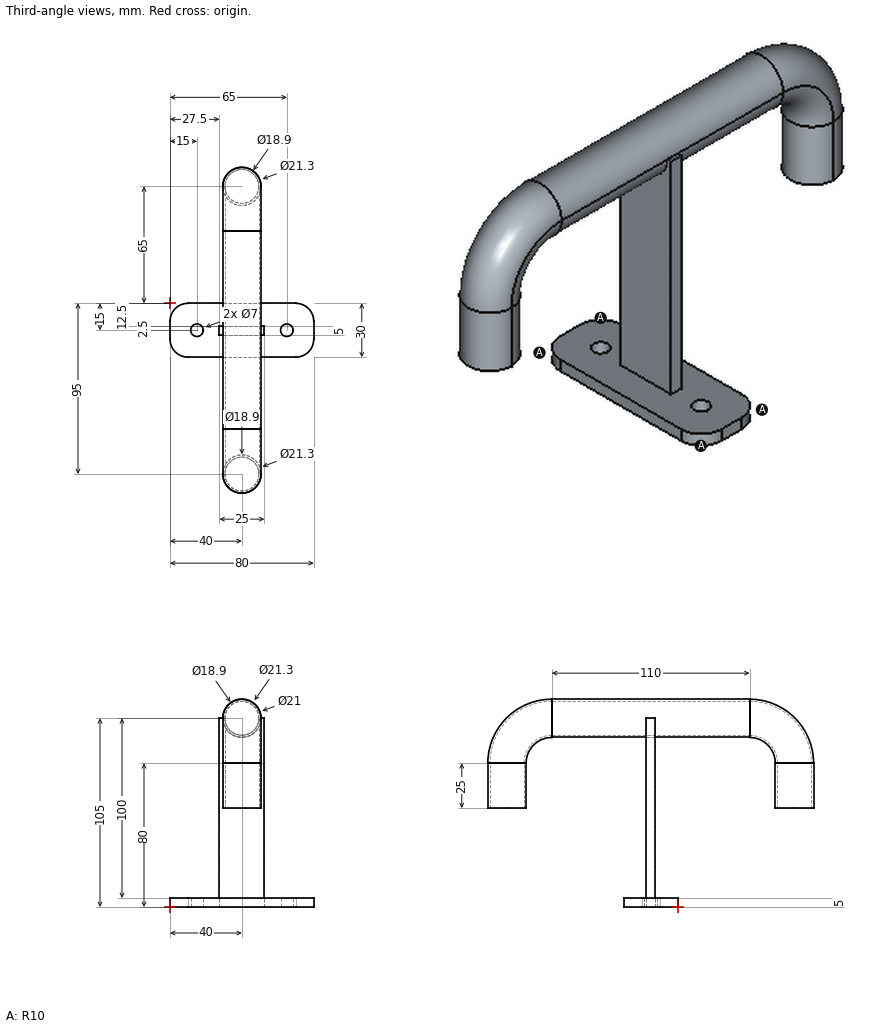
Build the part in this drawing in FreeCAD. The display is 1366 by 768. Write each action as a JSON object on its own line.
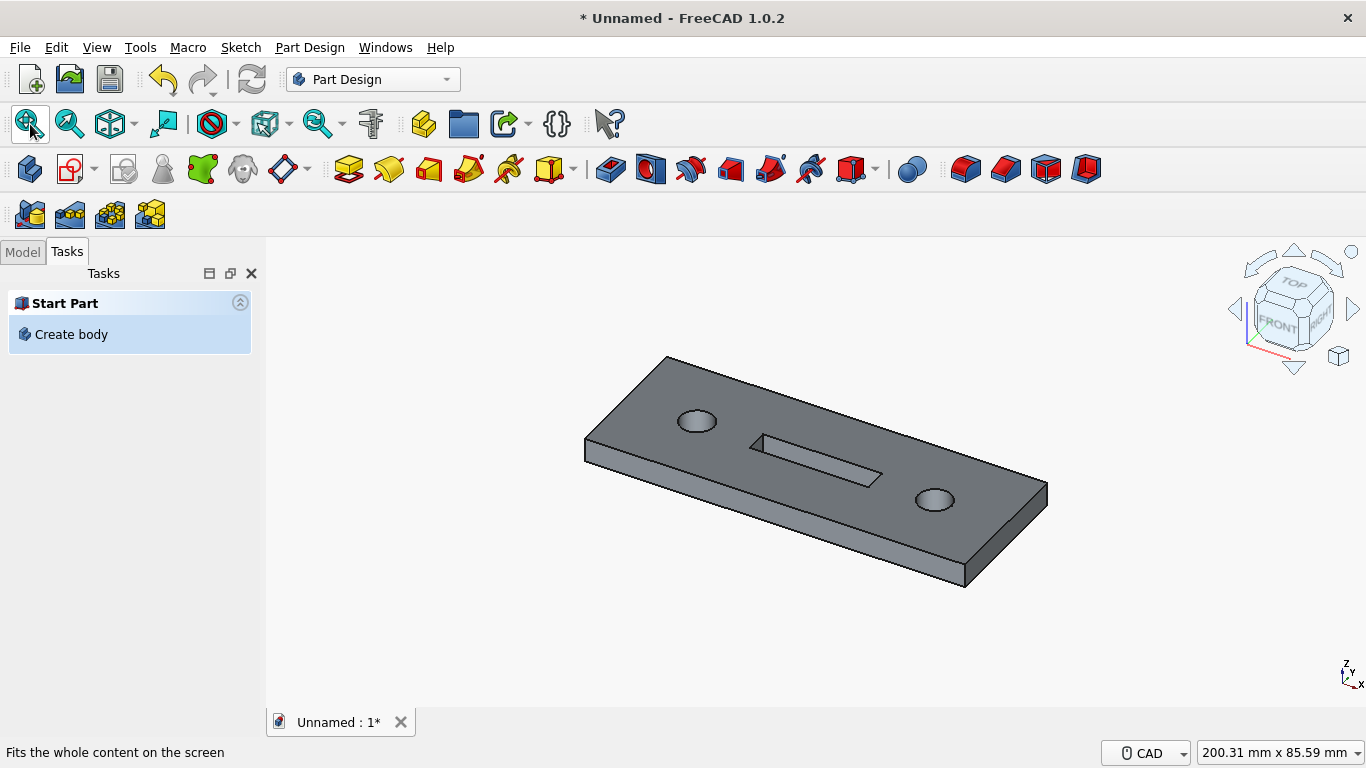
{"action": "left_click", "coordinate": [965, 575]}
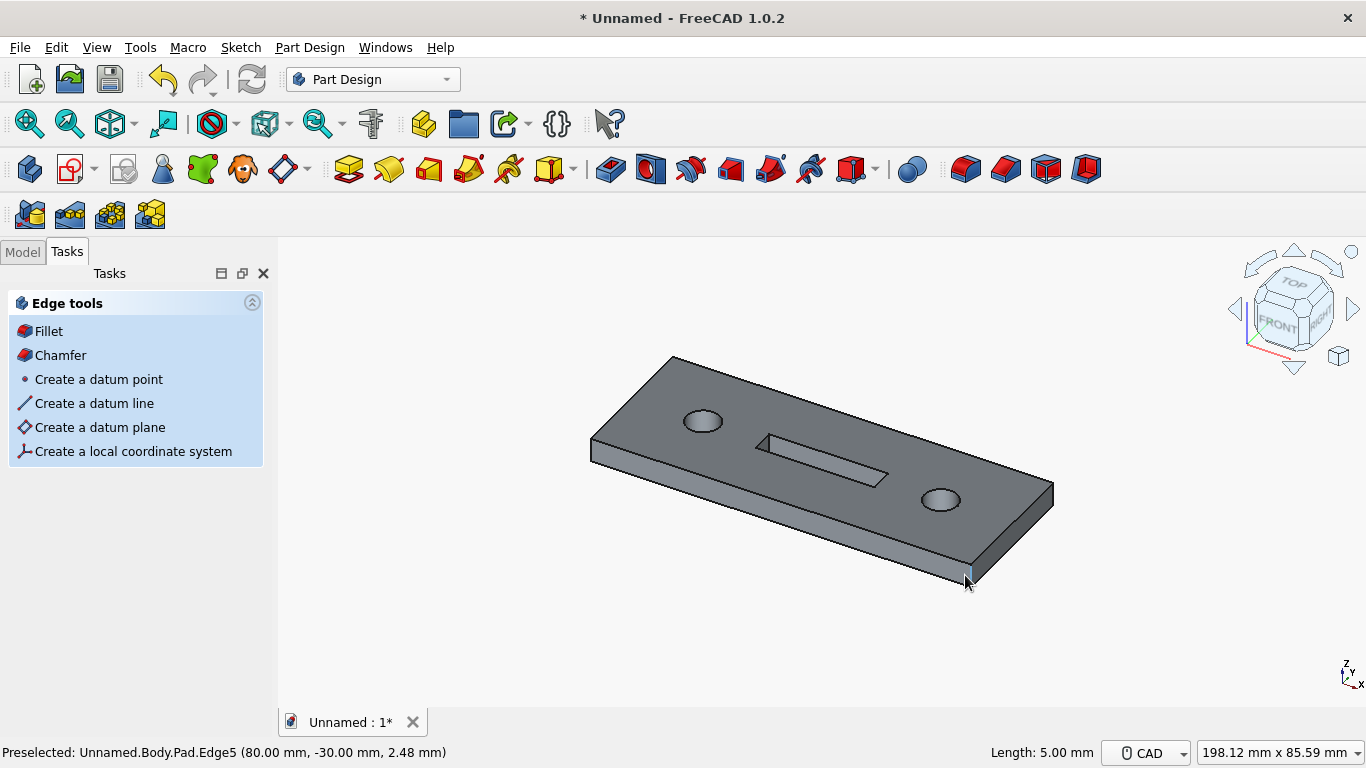
{"action": "key", "text": "0"}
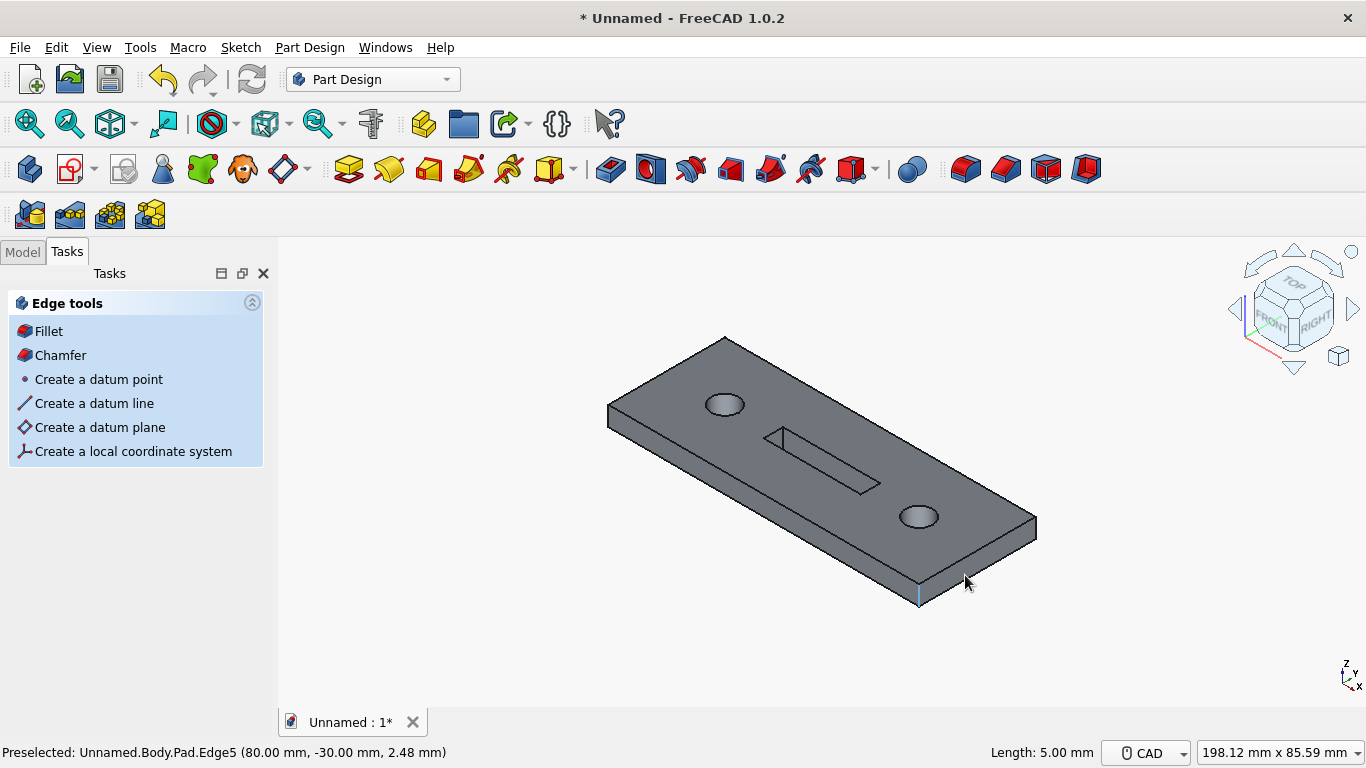
{"action": "key", "text": "2"}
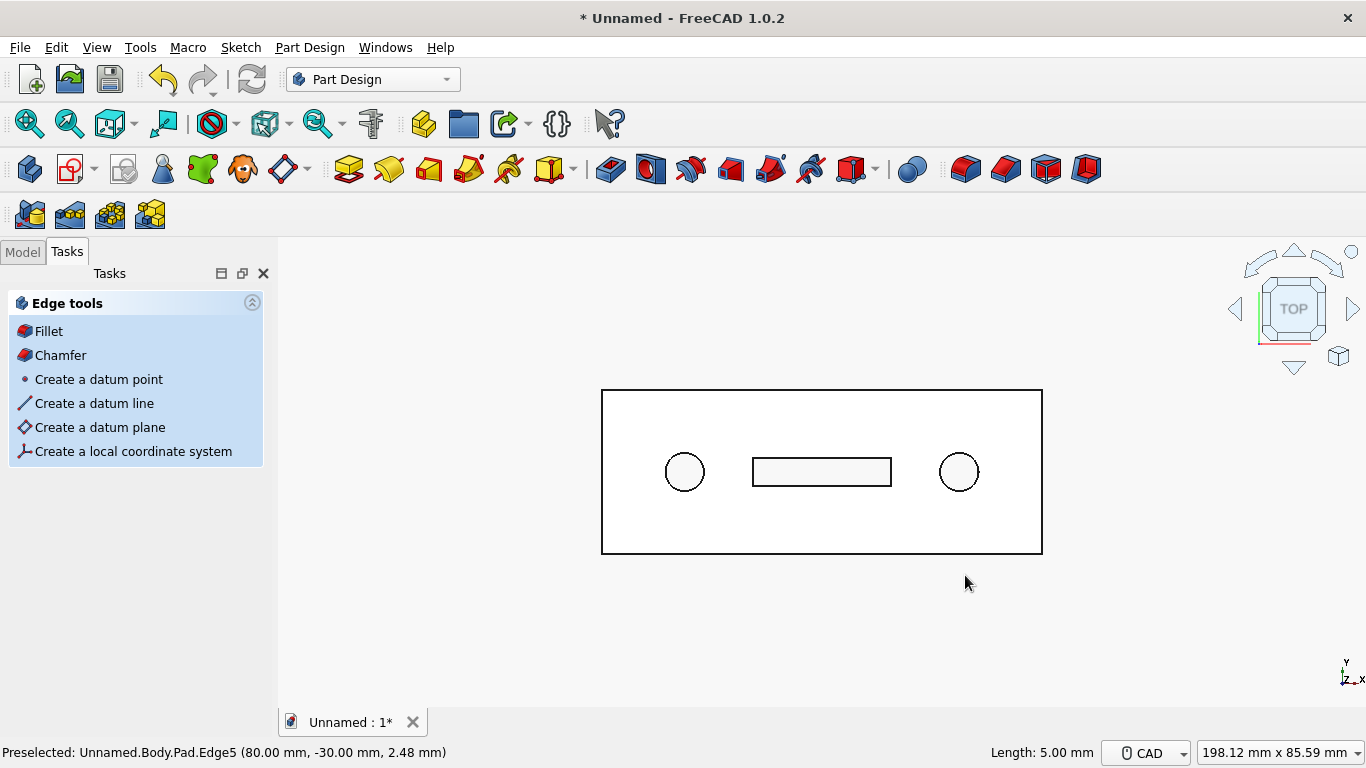
{"action": "left_click", "coordinate": [30, 124]}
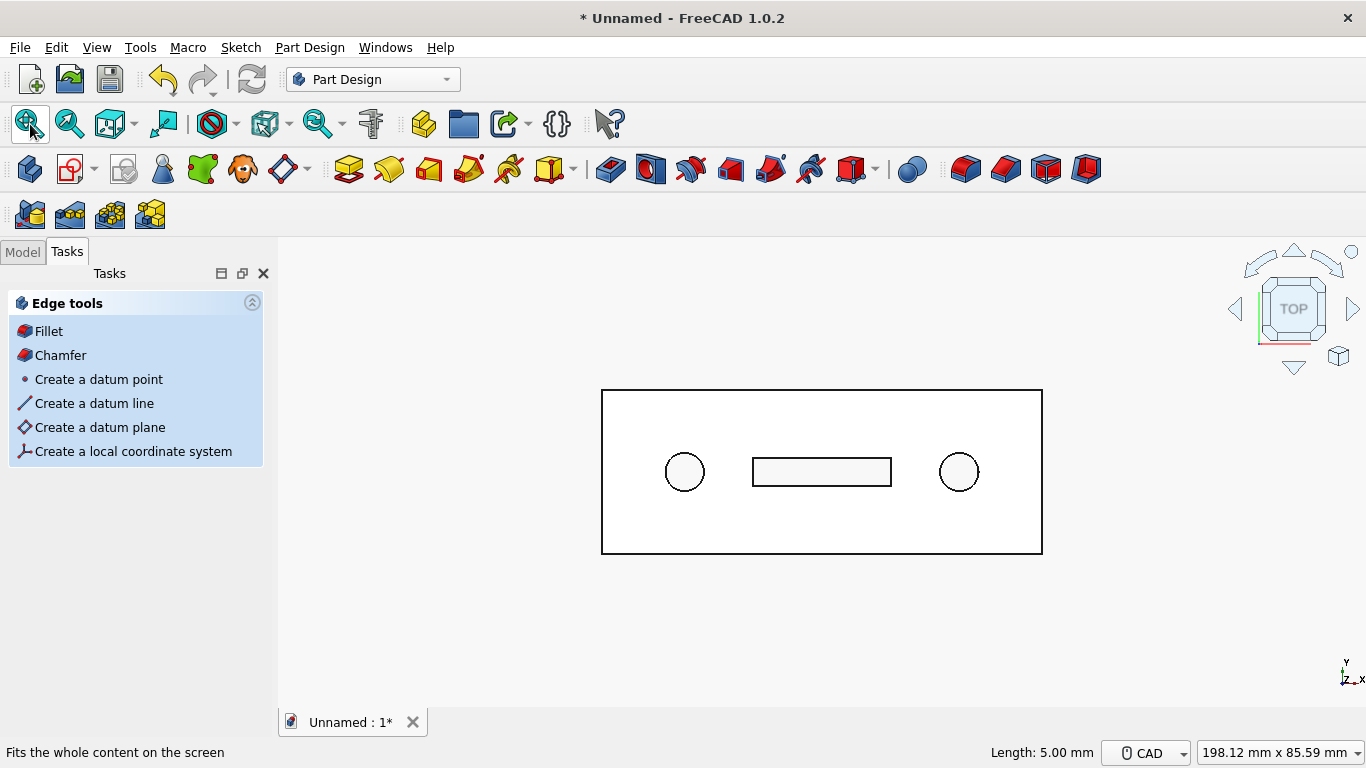
{"action": "key", "text": "1"}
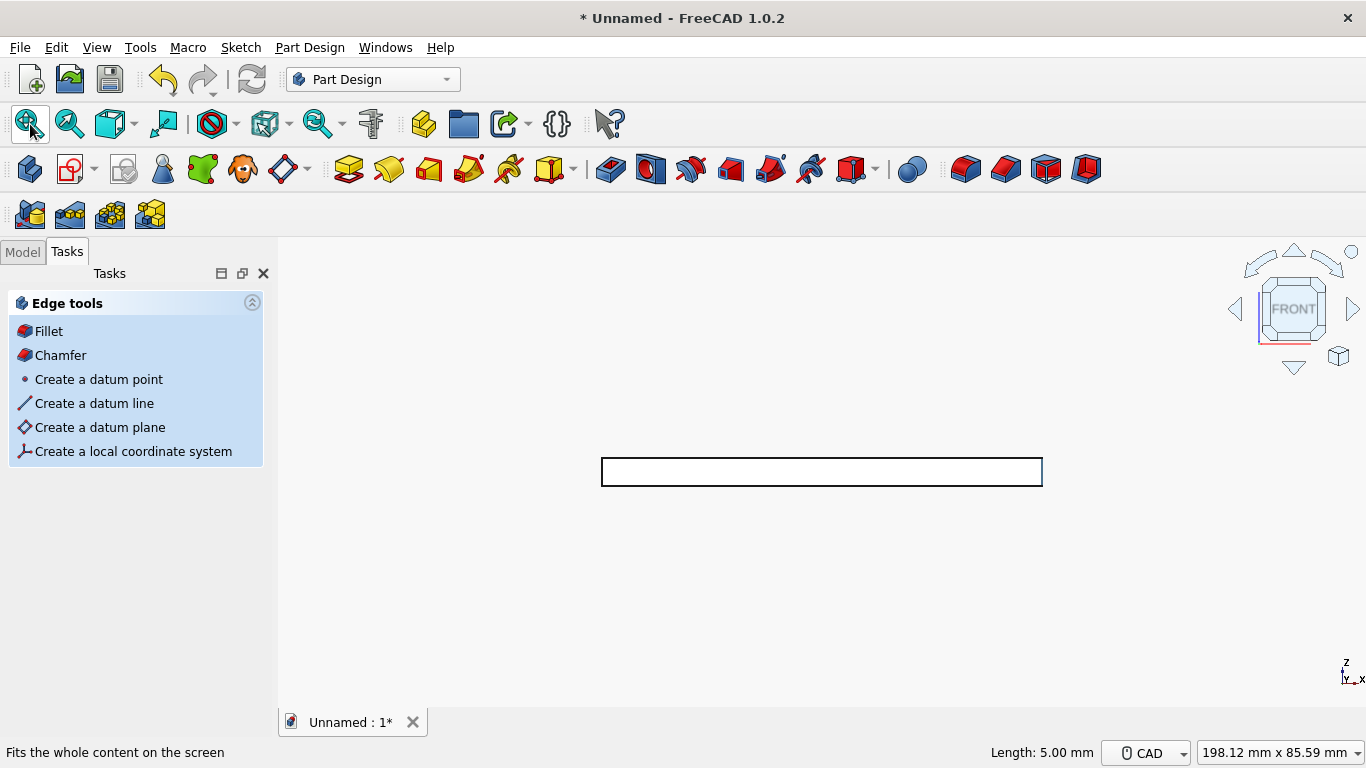
{"action": "left_click", "coordinate": [30, 124]}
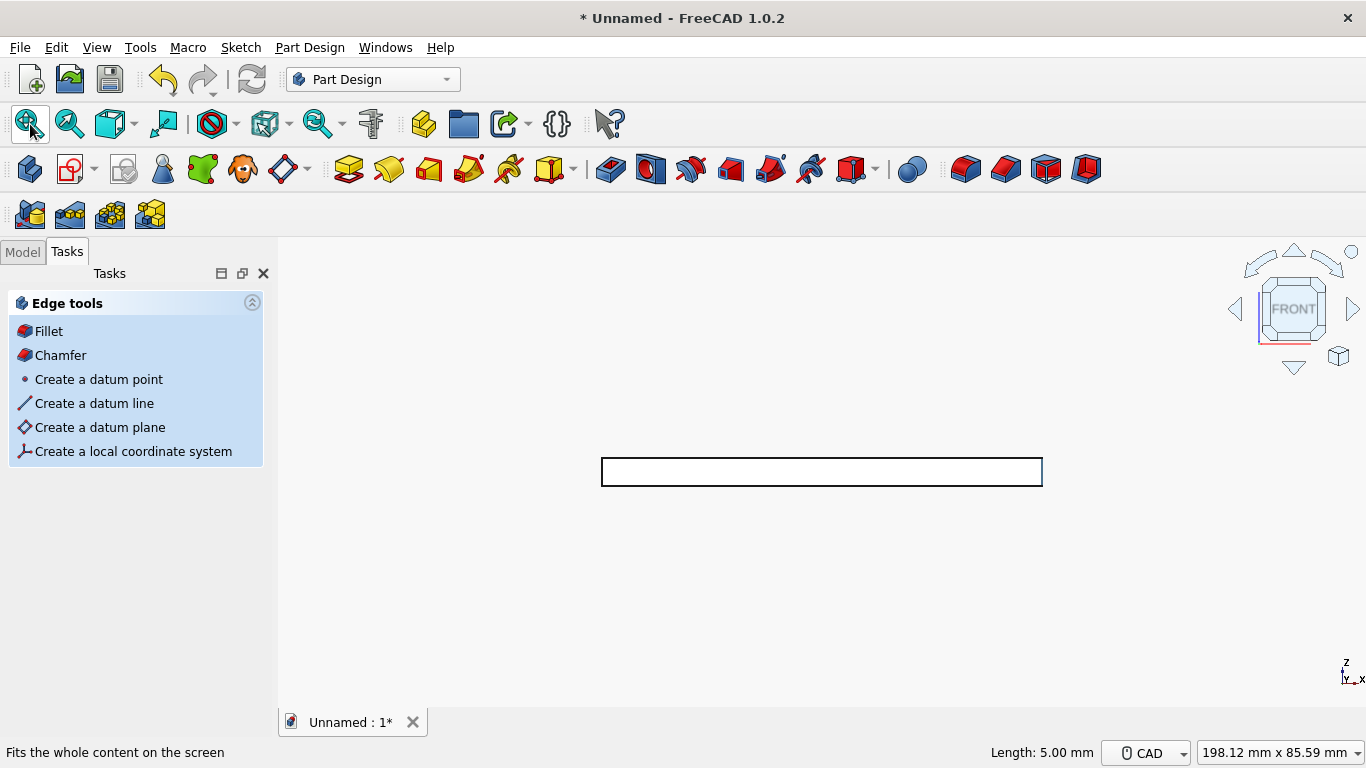
{"action": "left_click", "coordinate": [602, 471], "text": "ctrl"}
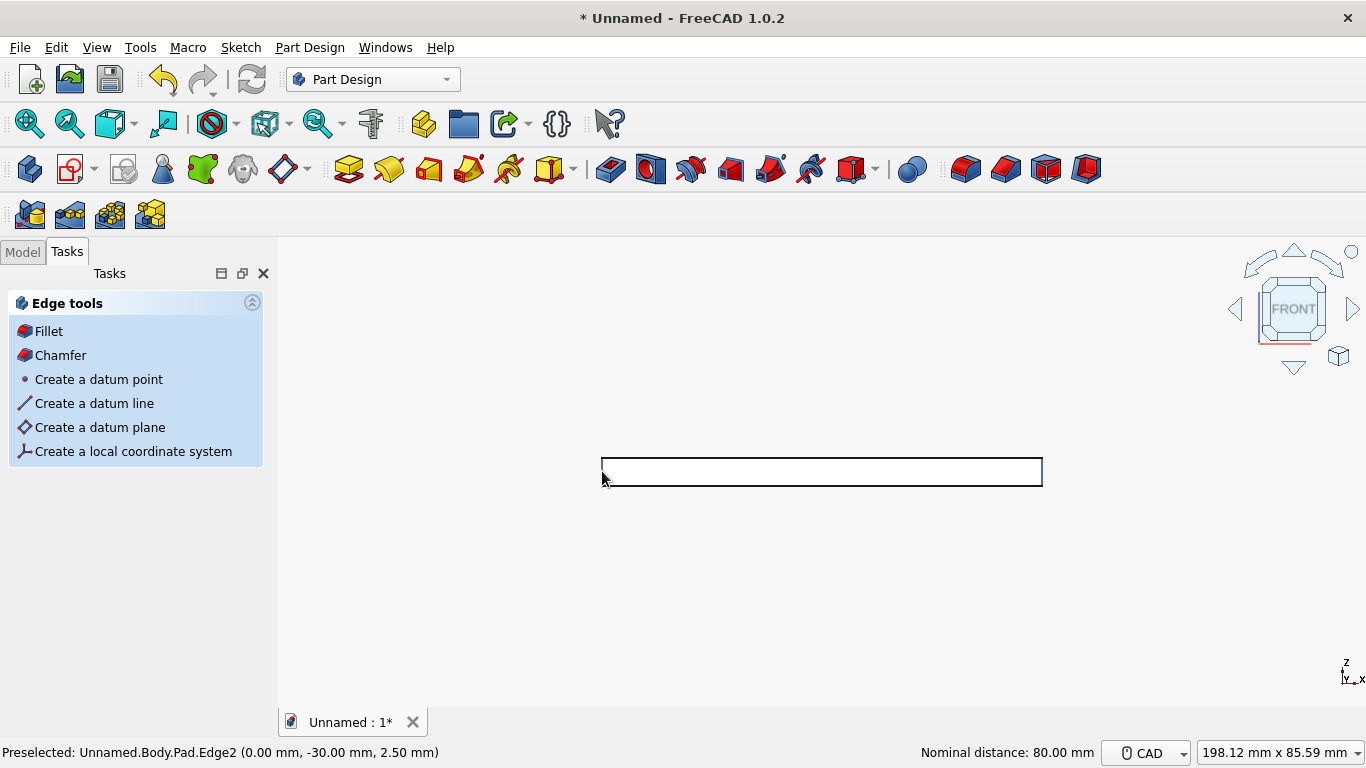
{"action": "key", "text": "3"}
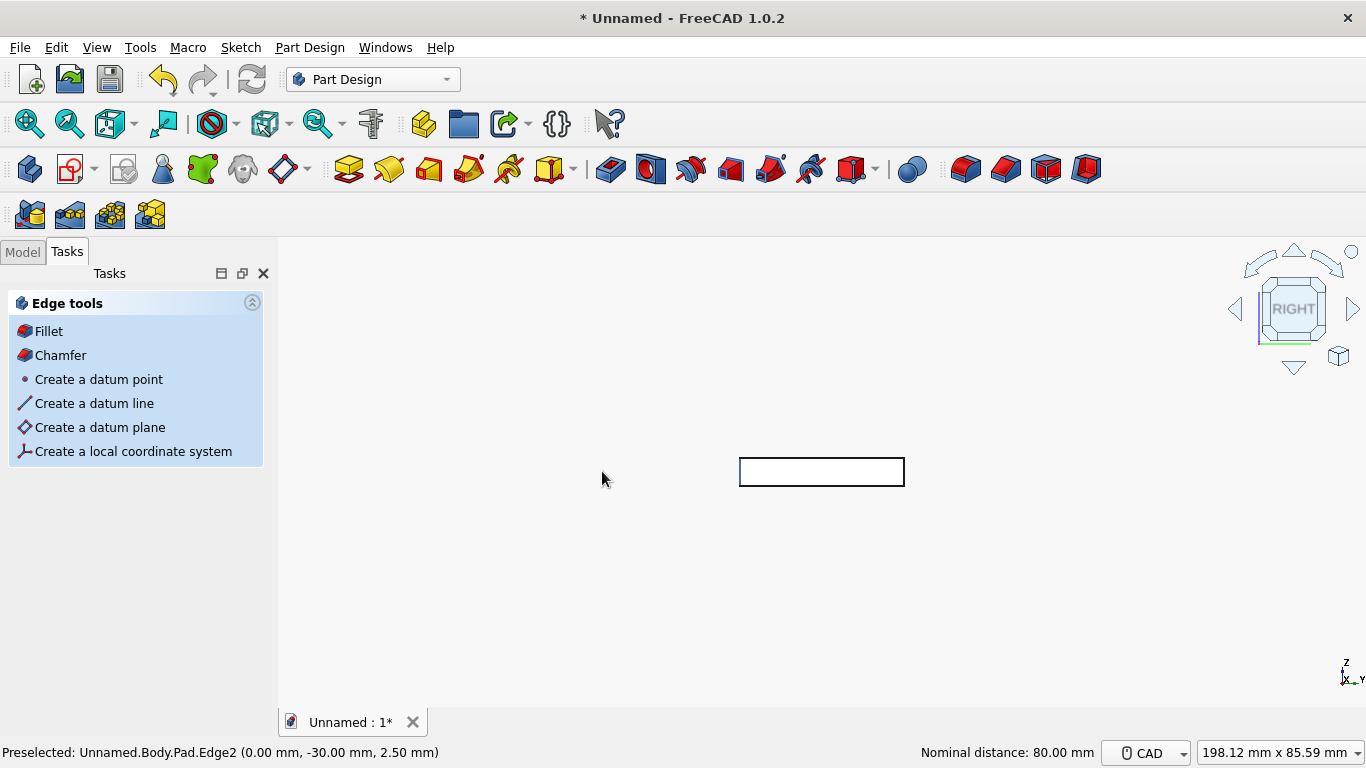
{"action": "left_click", "coordinate": [30, 124]}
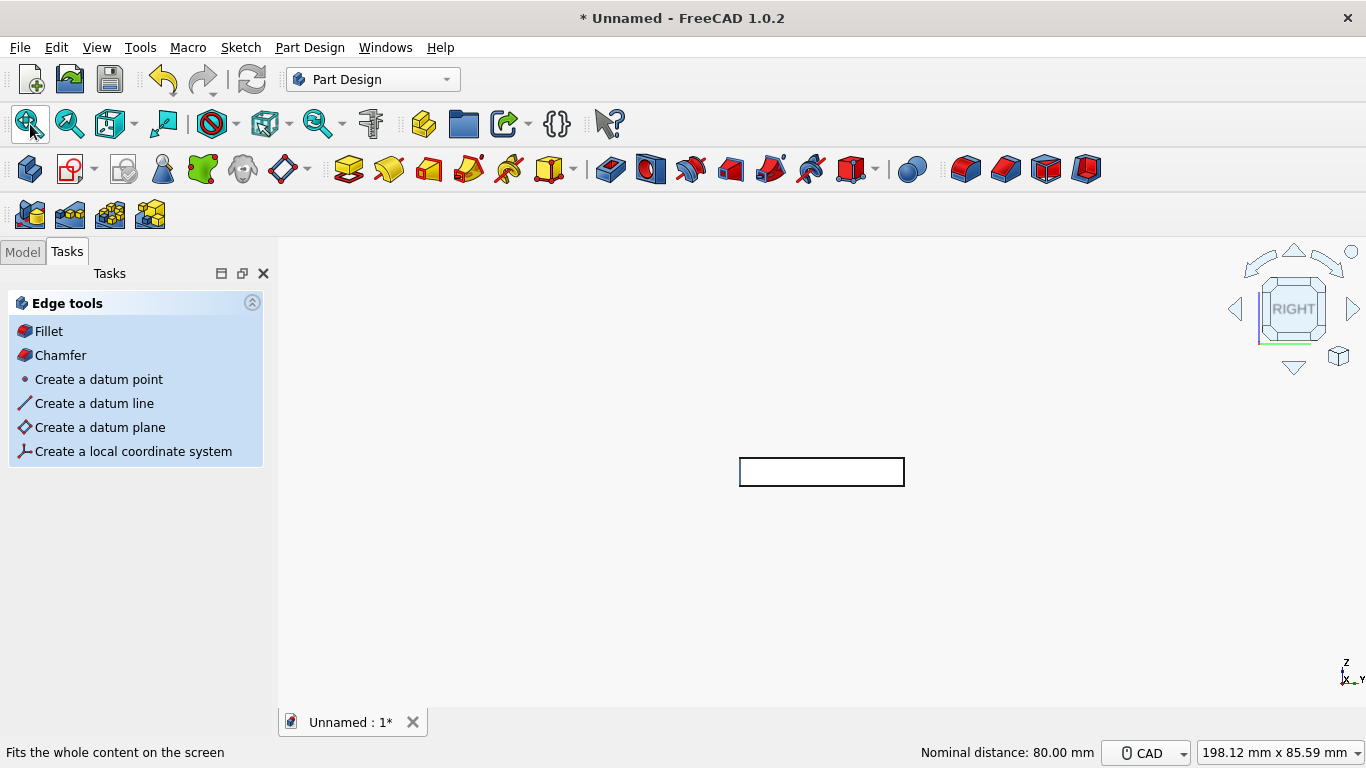
{"action": "left_click", "coordinate": [904, 471], "text": "ctrl"}